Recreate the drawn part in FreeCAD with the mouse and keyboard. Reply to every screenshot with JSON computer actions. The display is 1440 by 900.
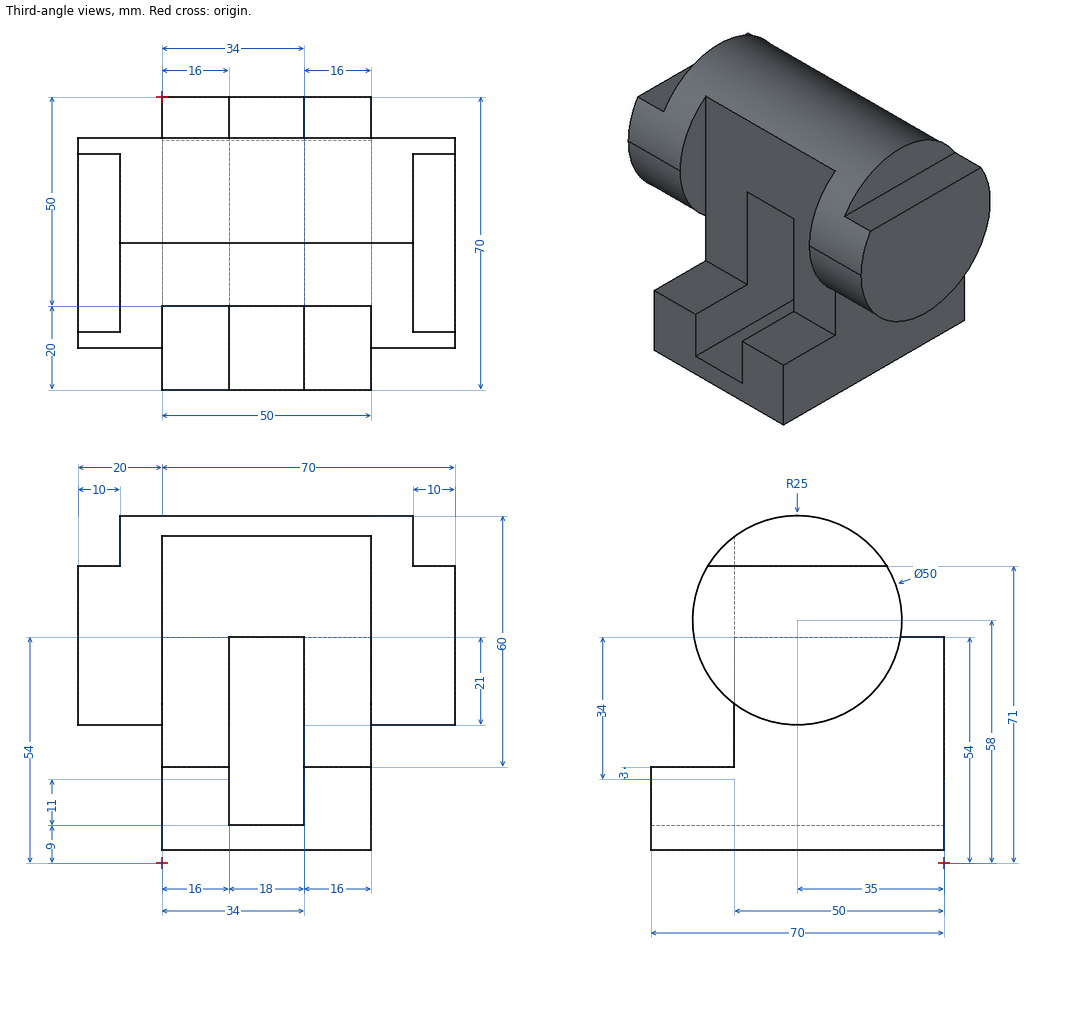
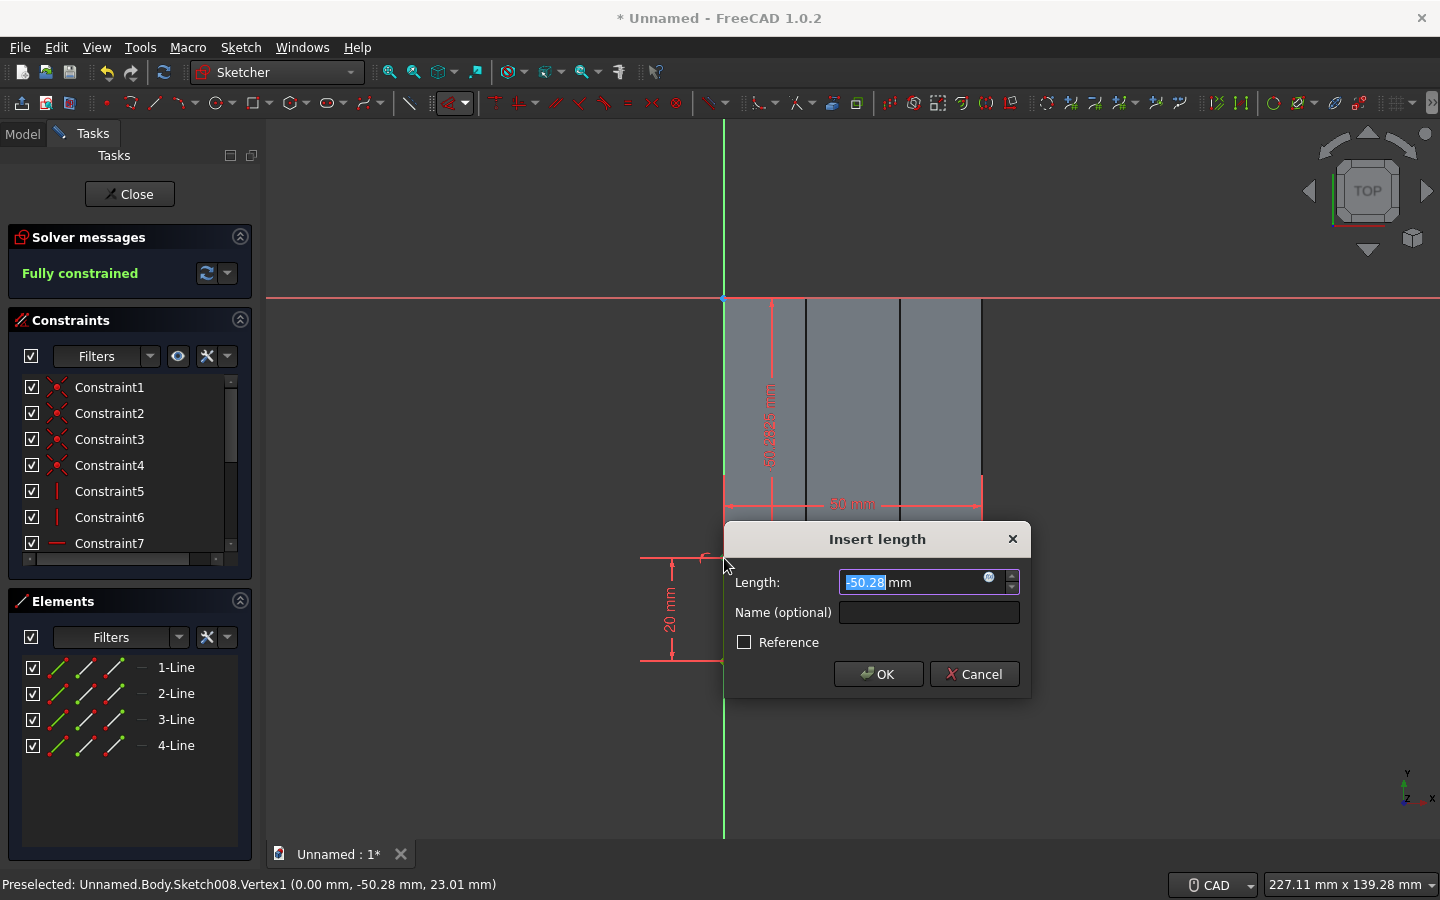
{"action": "type", "text": "-50"}
{"action": "key", "text": "Return"}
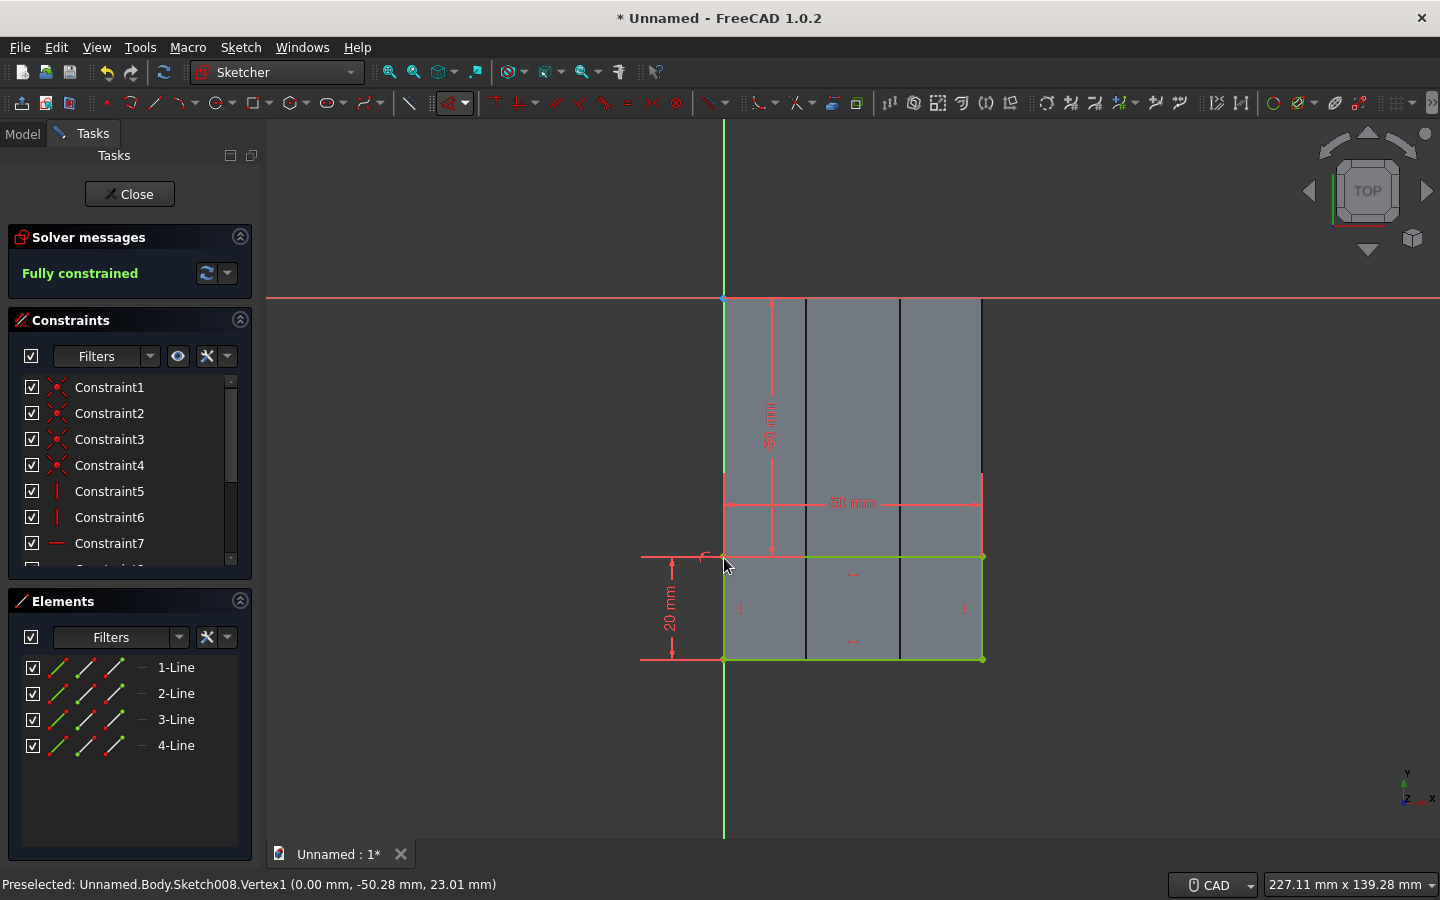
{"action": "left_click", "coordinate": [130, 194]}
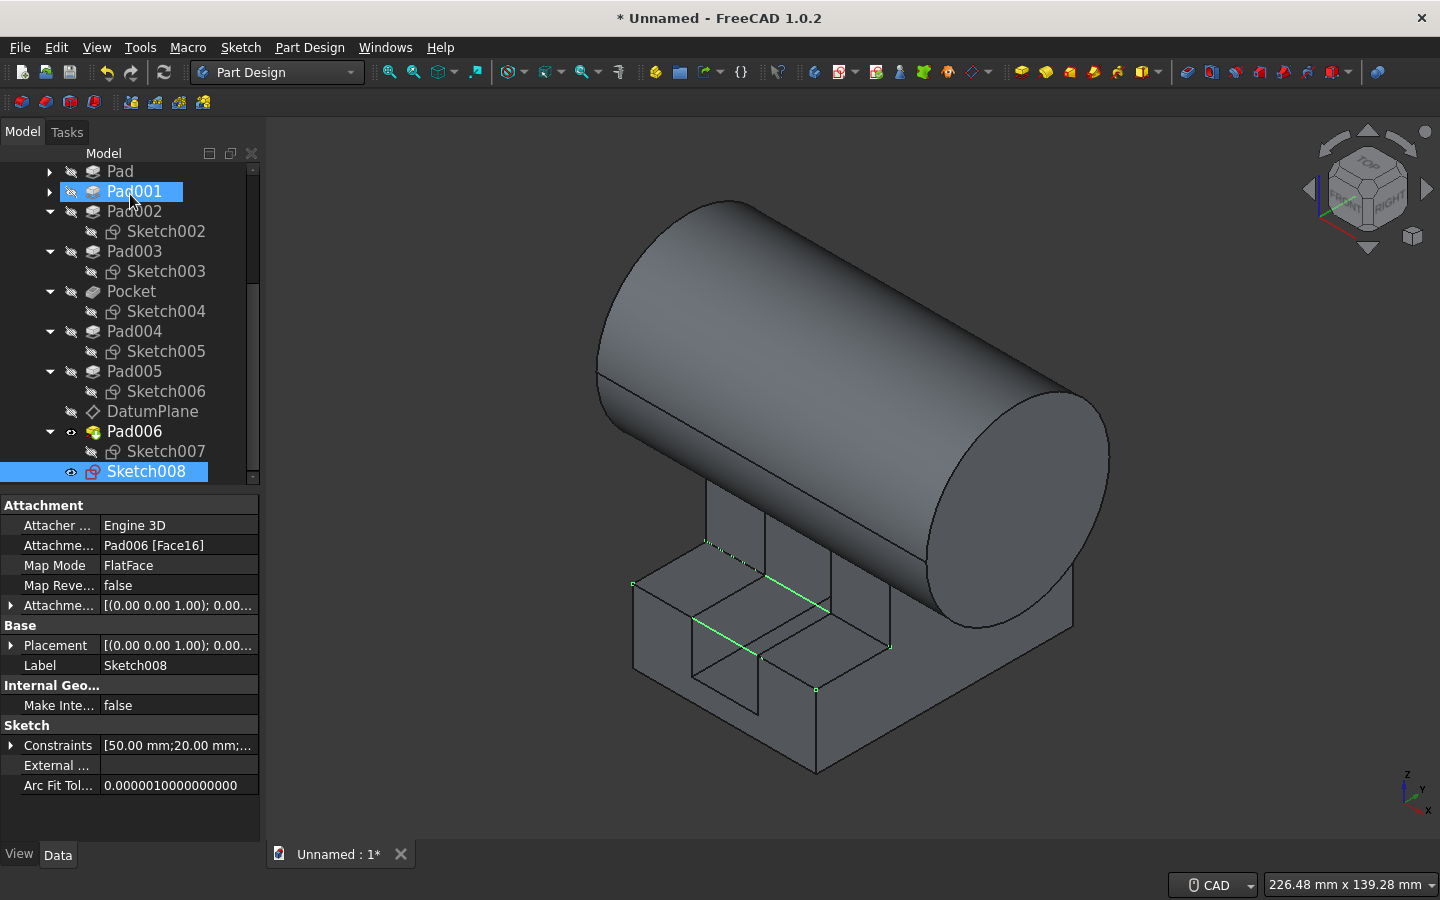
{"action": "left_click", "coordinate": [1188, 72]}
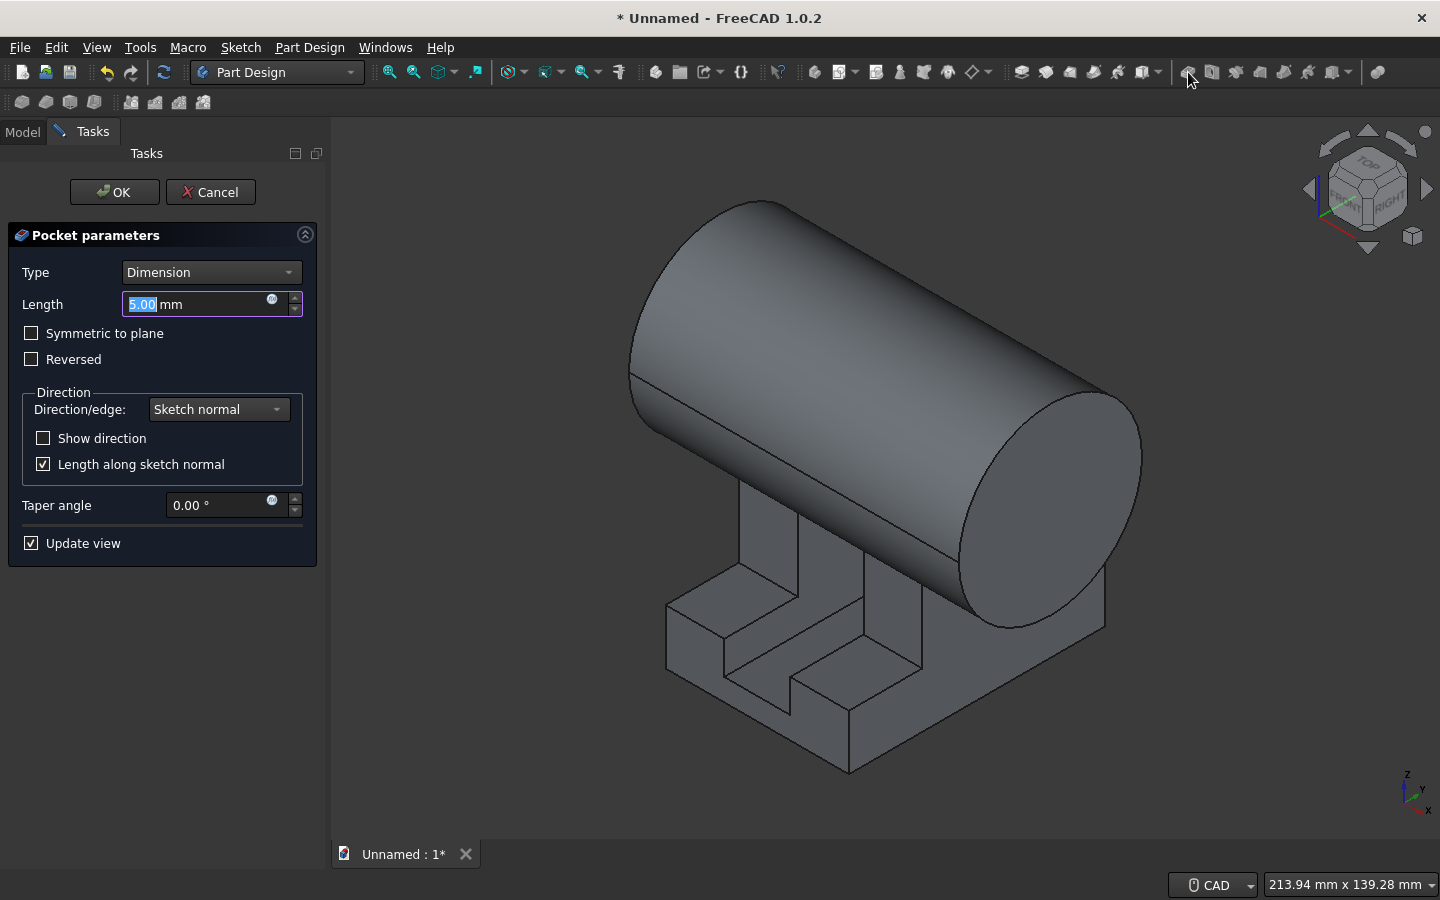
{"action": "type", "text": "60"}
{"action": "key", "text": "Tab"}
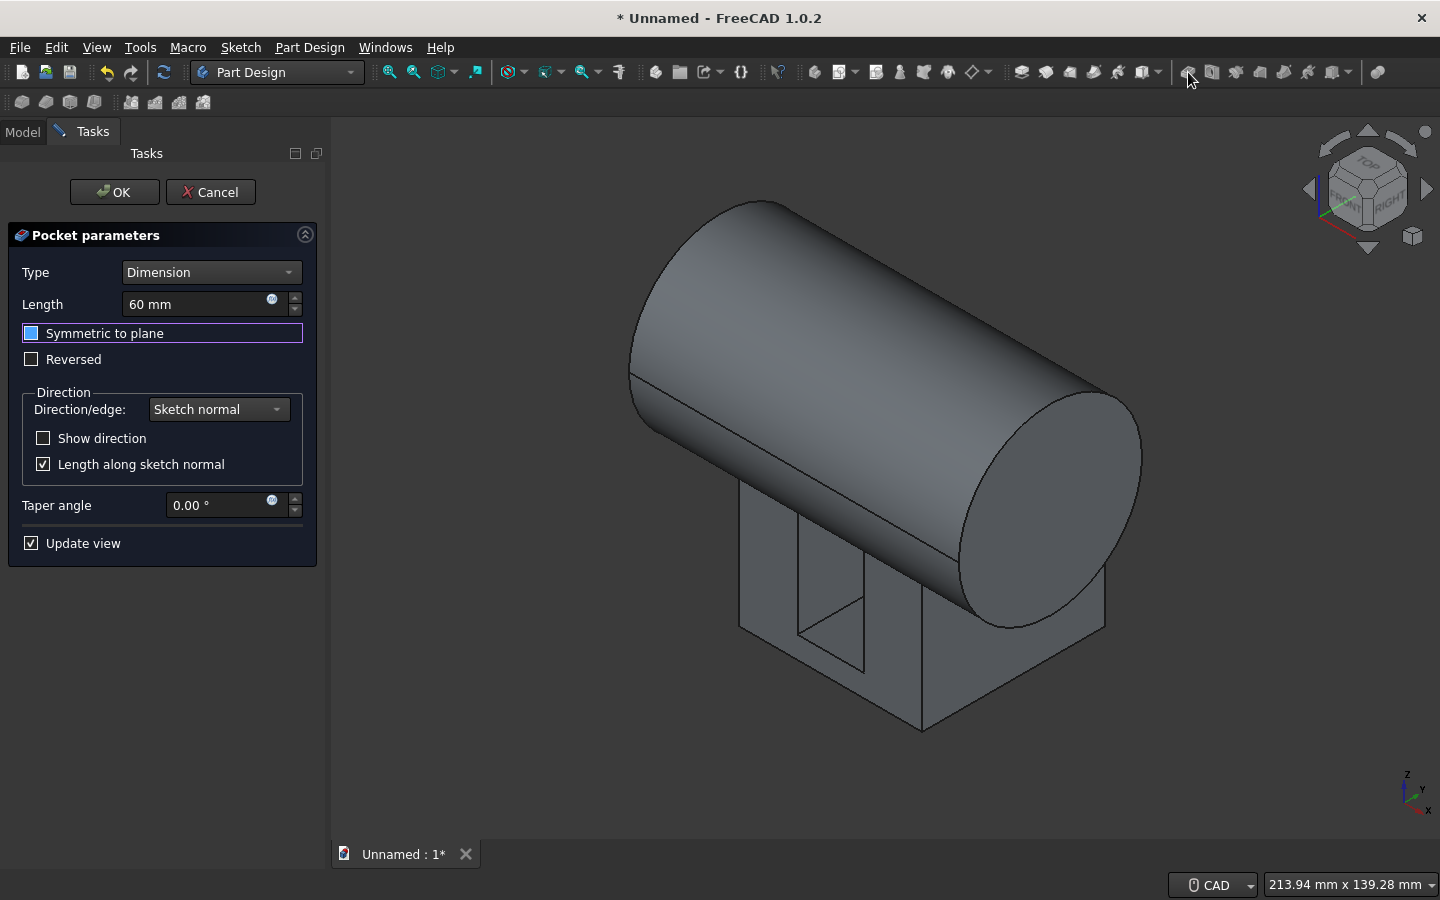
{"action": "left_click", "coordinate": [30, 359]}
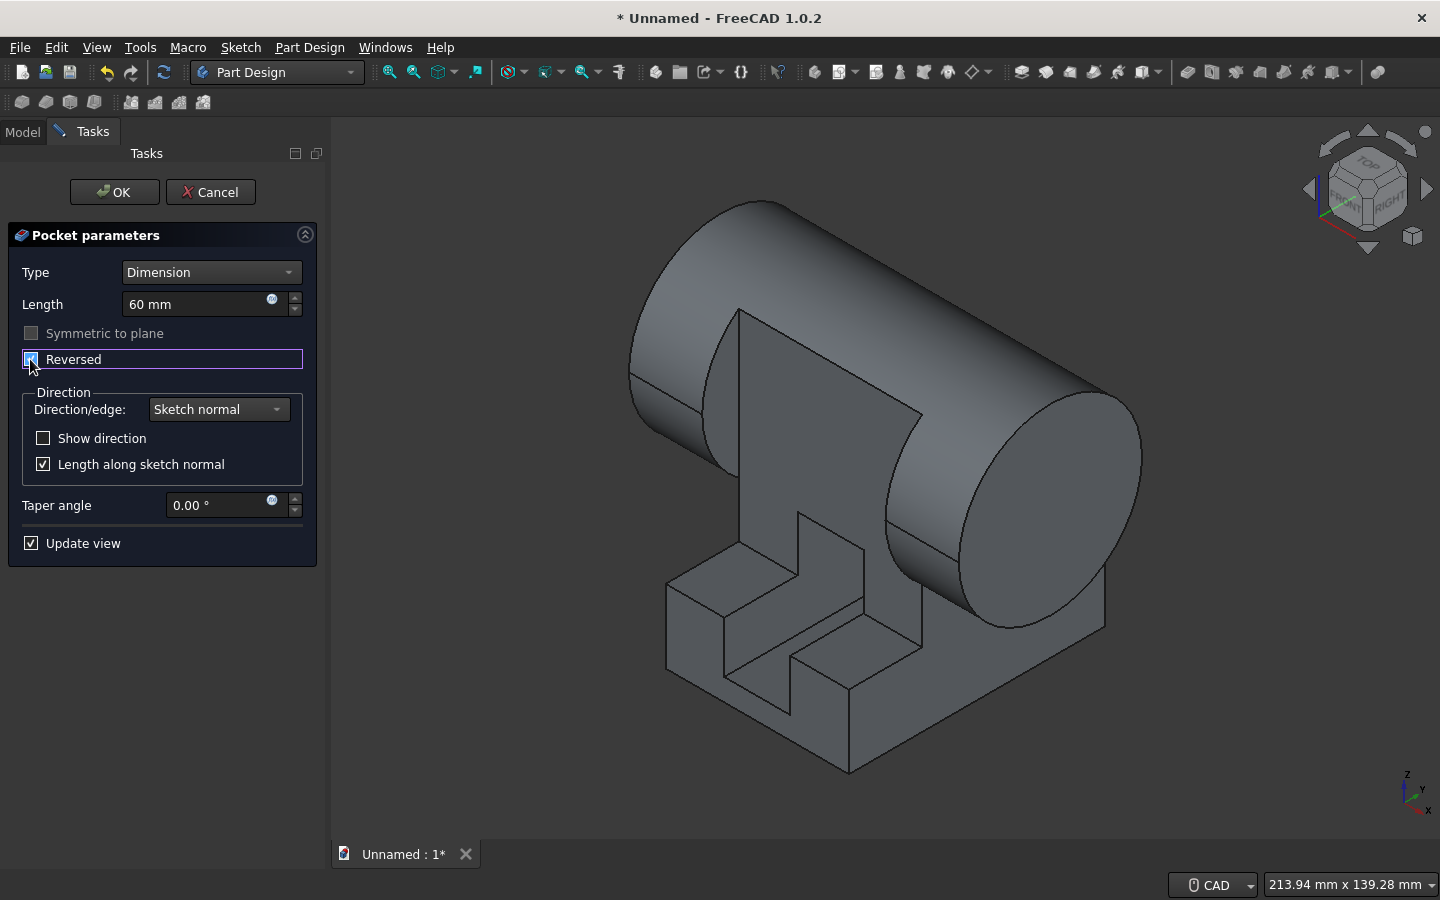
{"action": "left_click", "coordinate": [115, 192]}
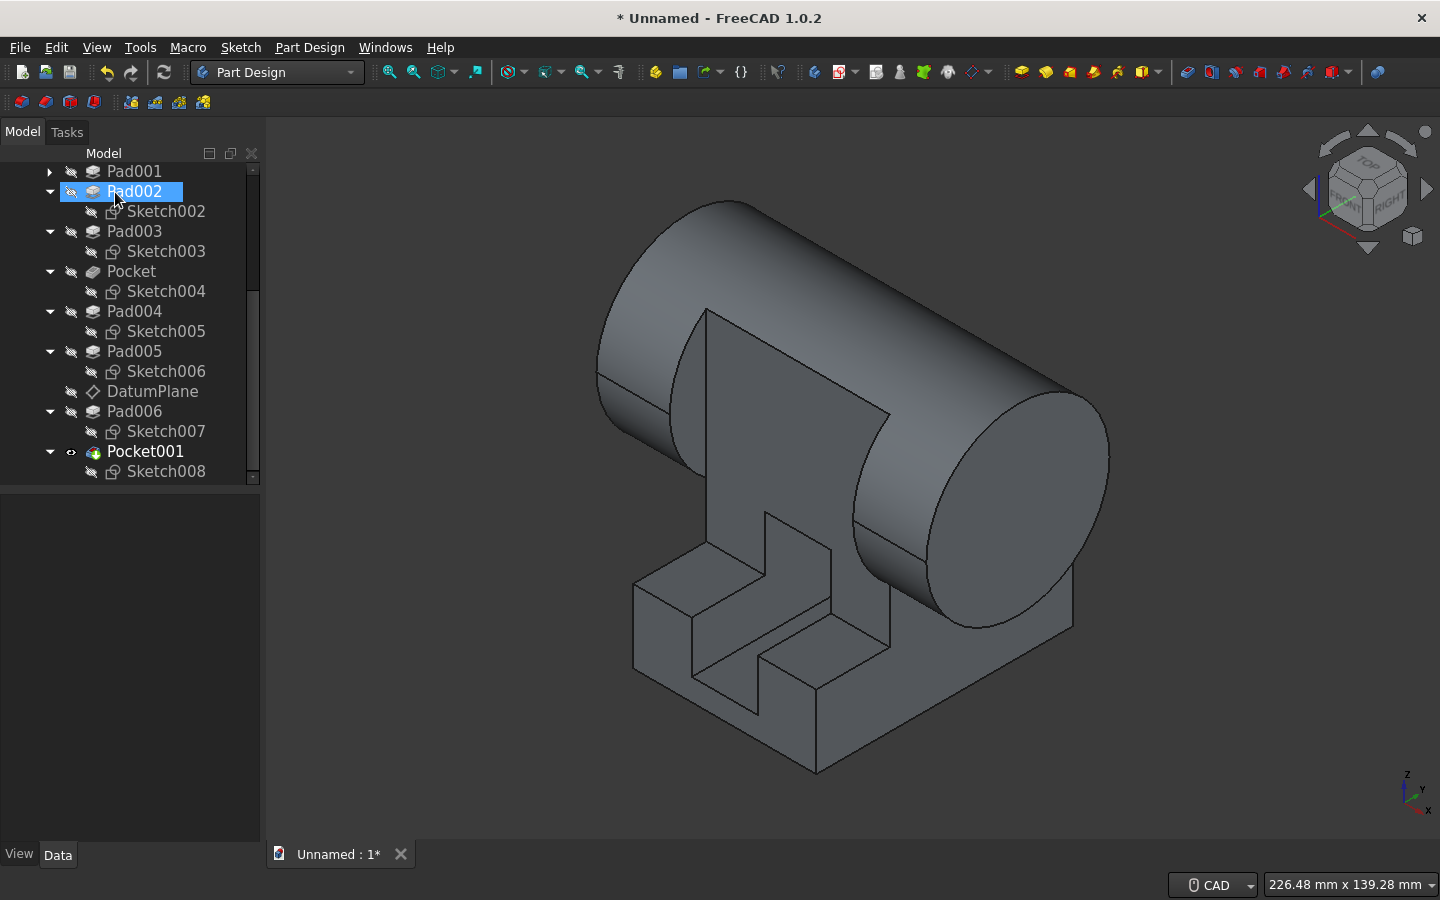
{"action": "left_click", "coordinate": [798, 444]}